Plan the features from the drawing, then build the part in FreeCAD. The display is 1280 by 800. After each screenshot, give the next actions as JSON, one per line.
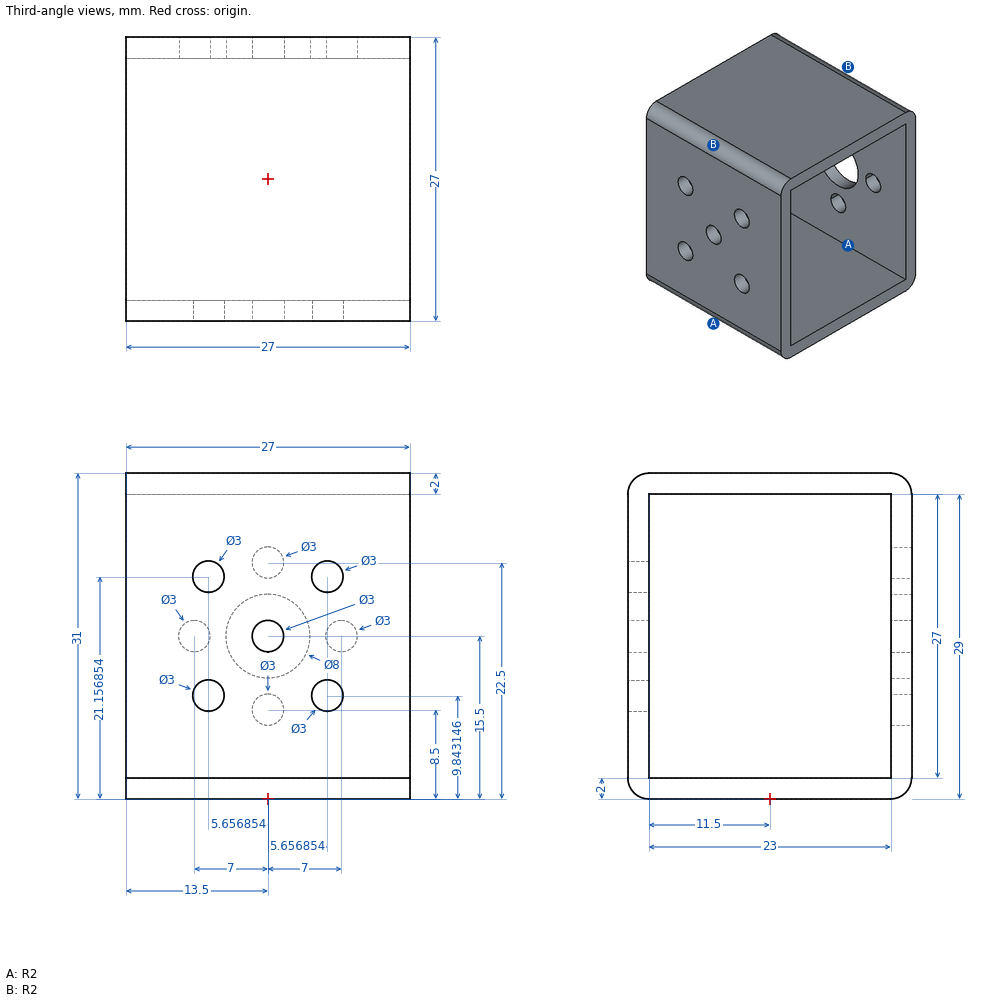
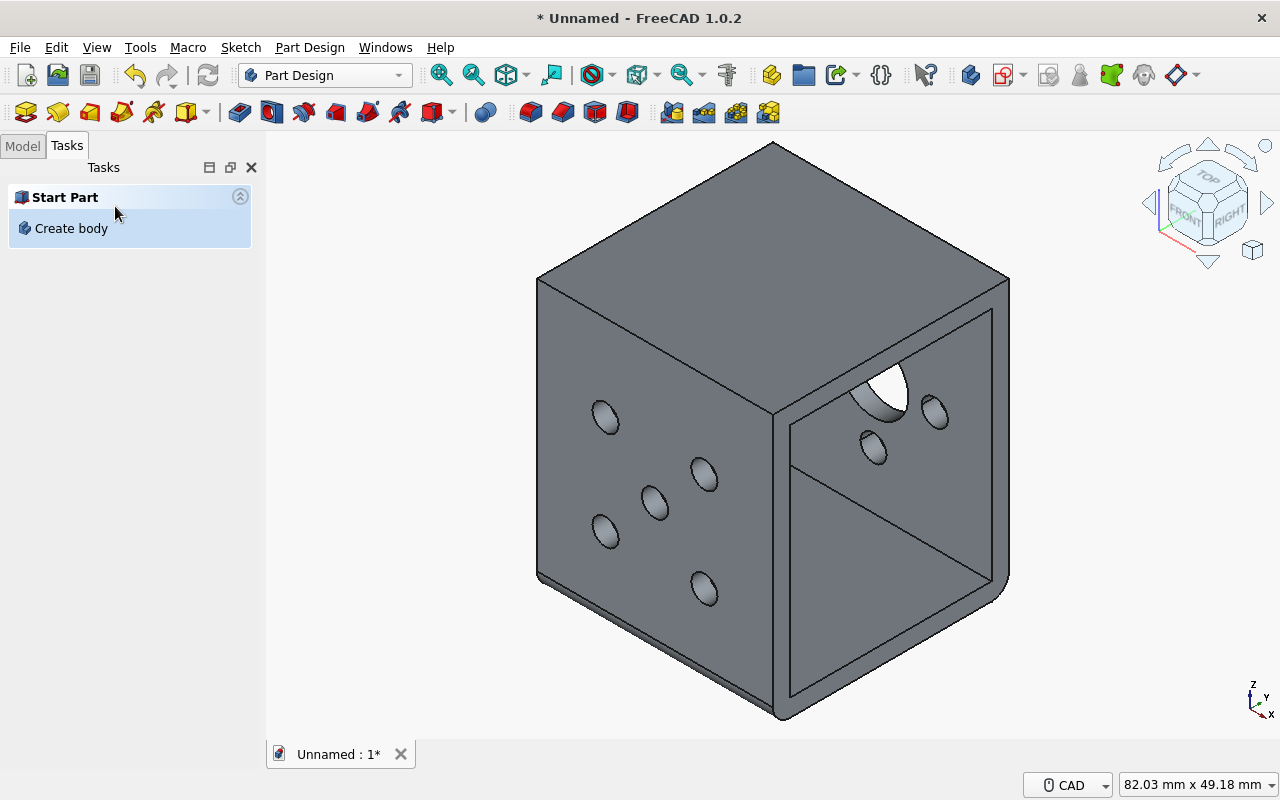
{"action": "left_click", "coordinate": [655, 346]}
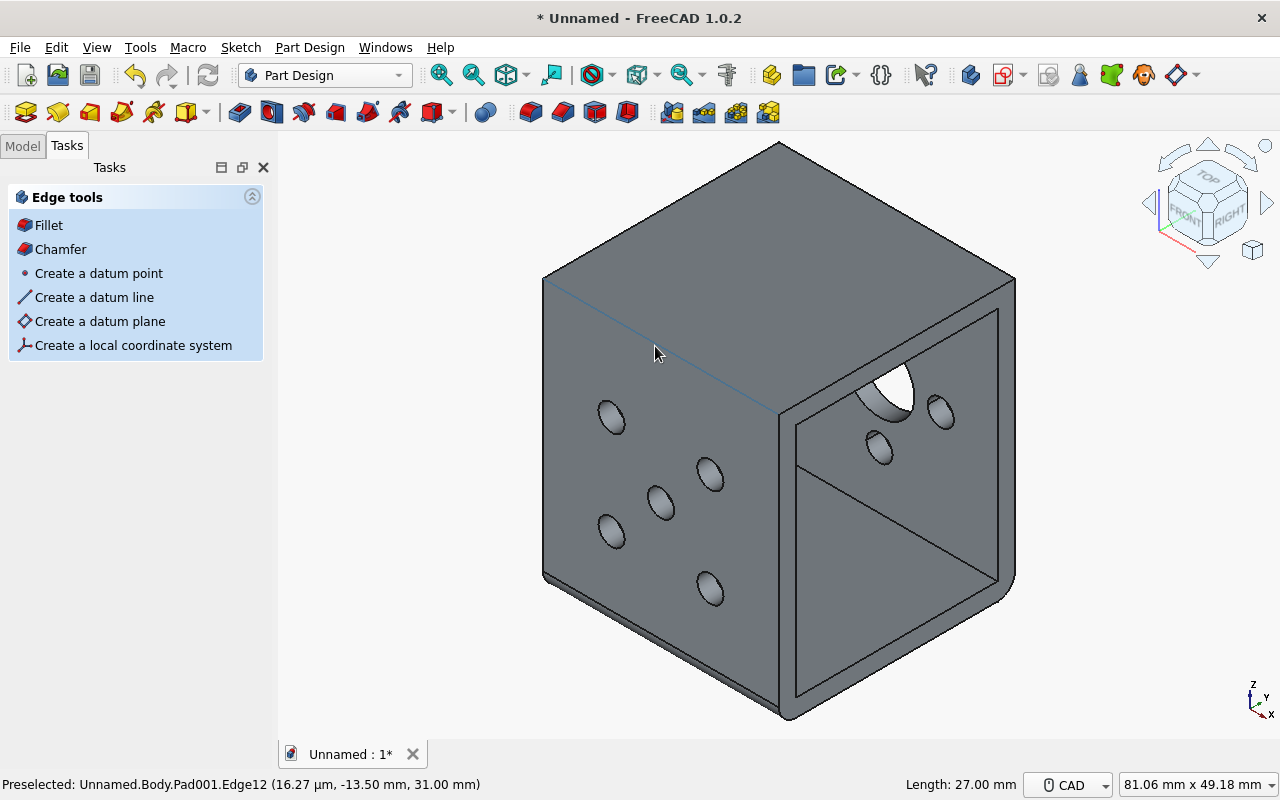
{"action": "key", "text": "2"}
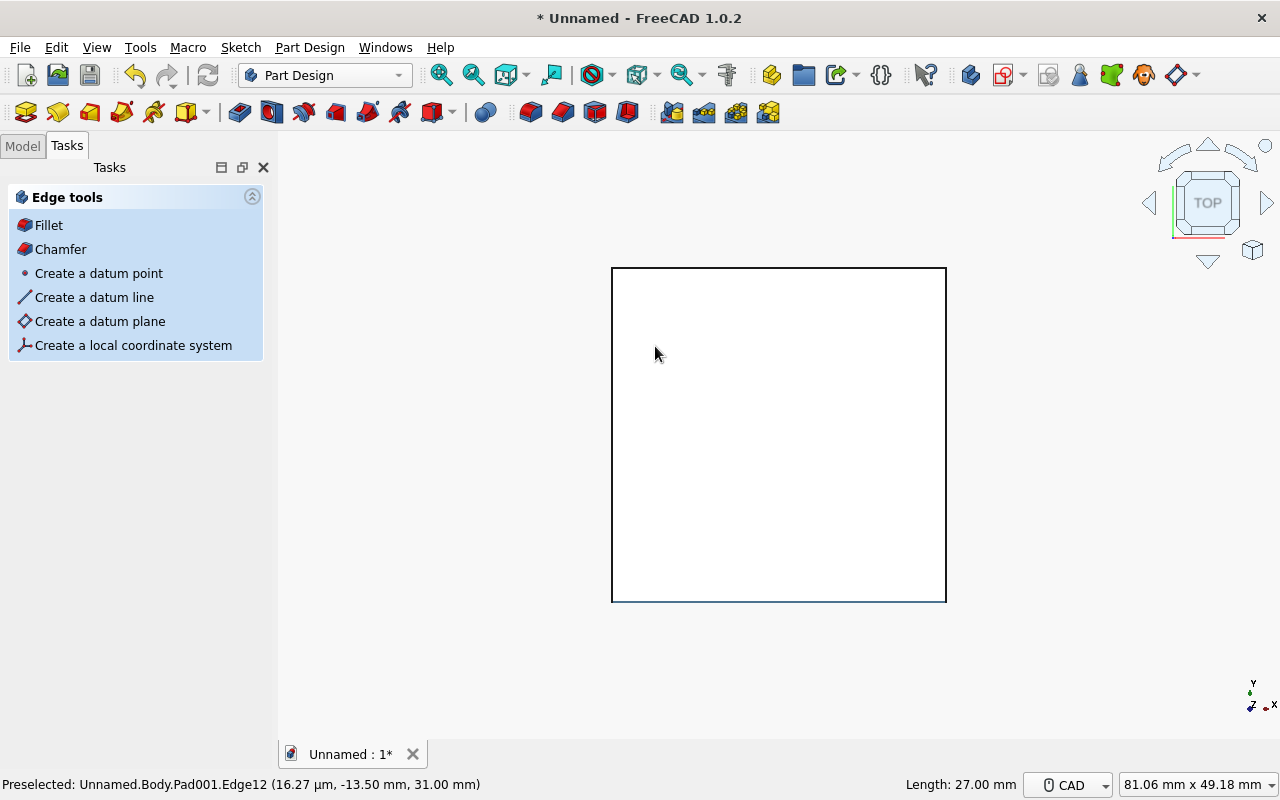
{"action": "left_click", "coordinate": [779, 267], "text": "ctrl"}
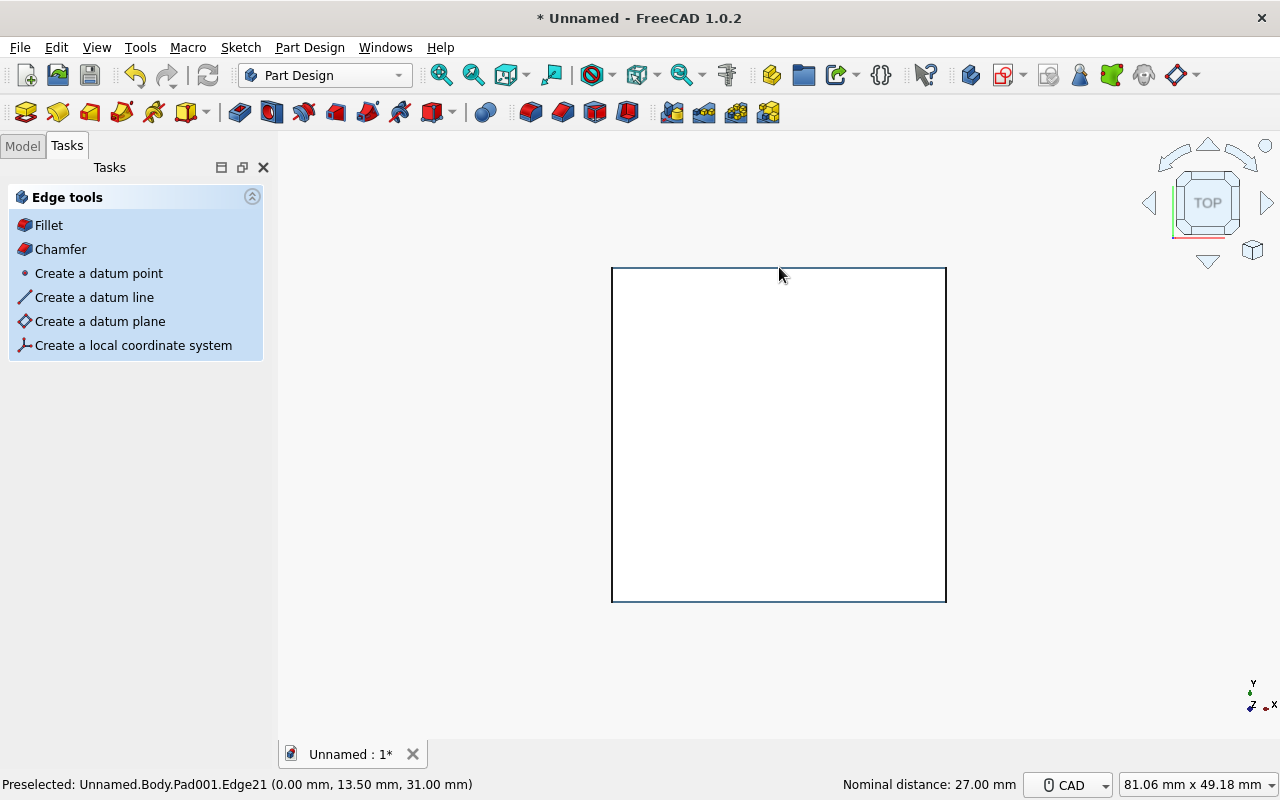
{"action": "left_click", "coordinate": [532, 112]}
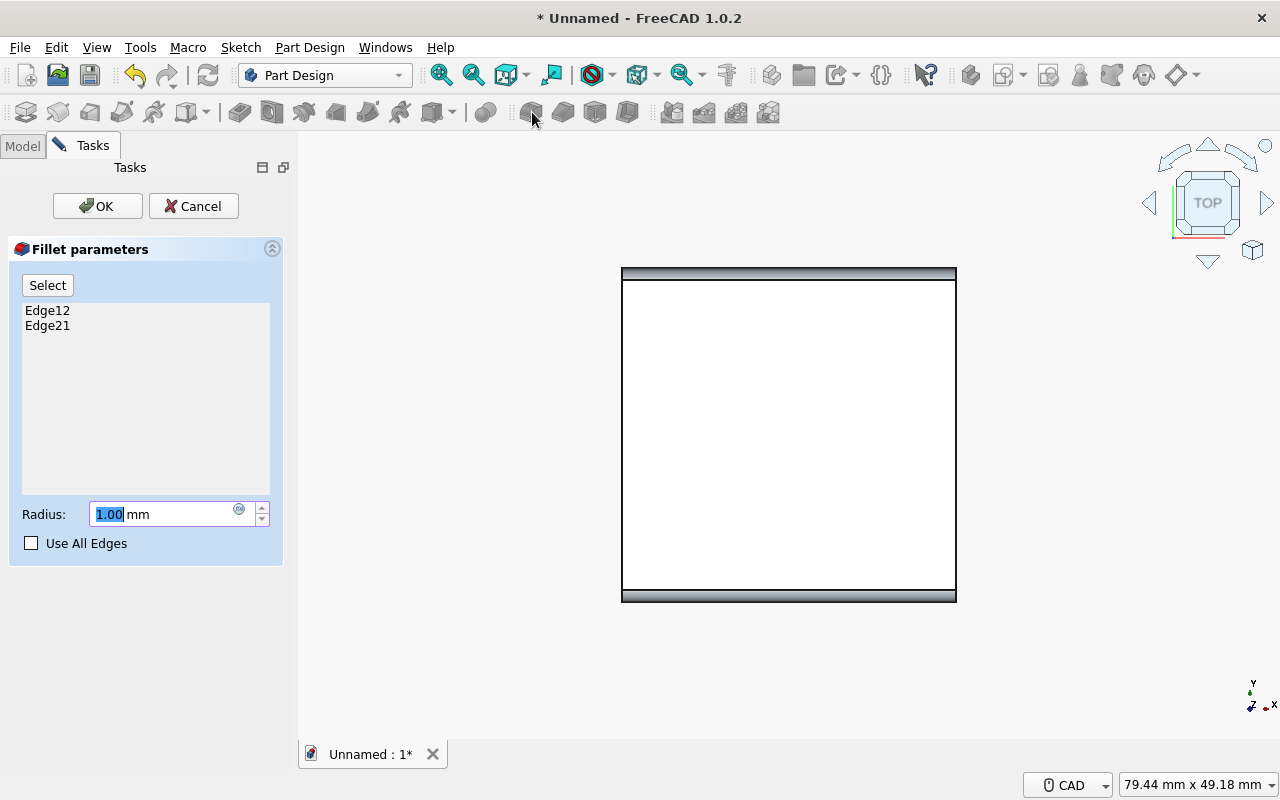
{"action": "type", "text": "2"}
{"action": "key", "text": "Tab"}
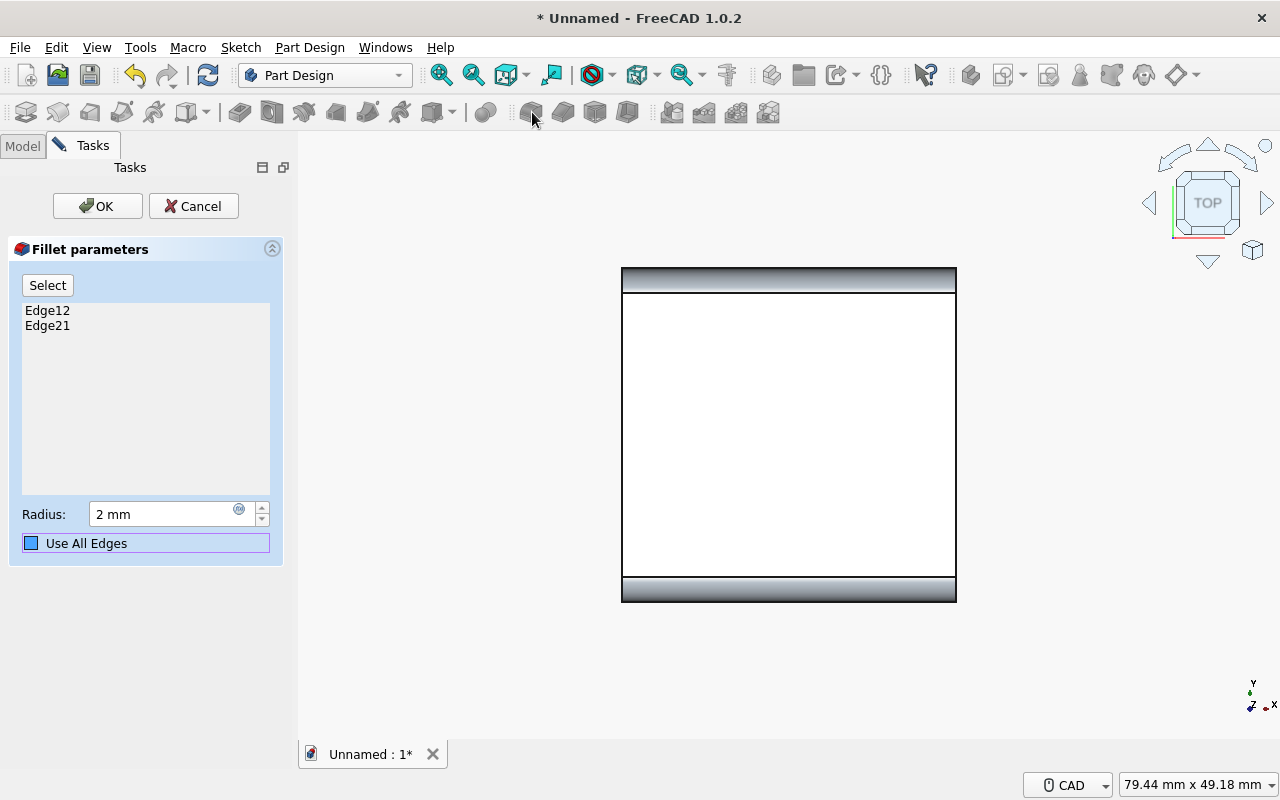
{"action": "left_click", "coordinate": [98, 206]}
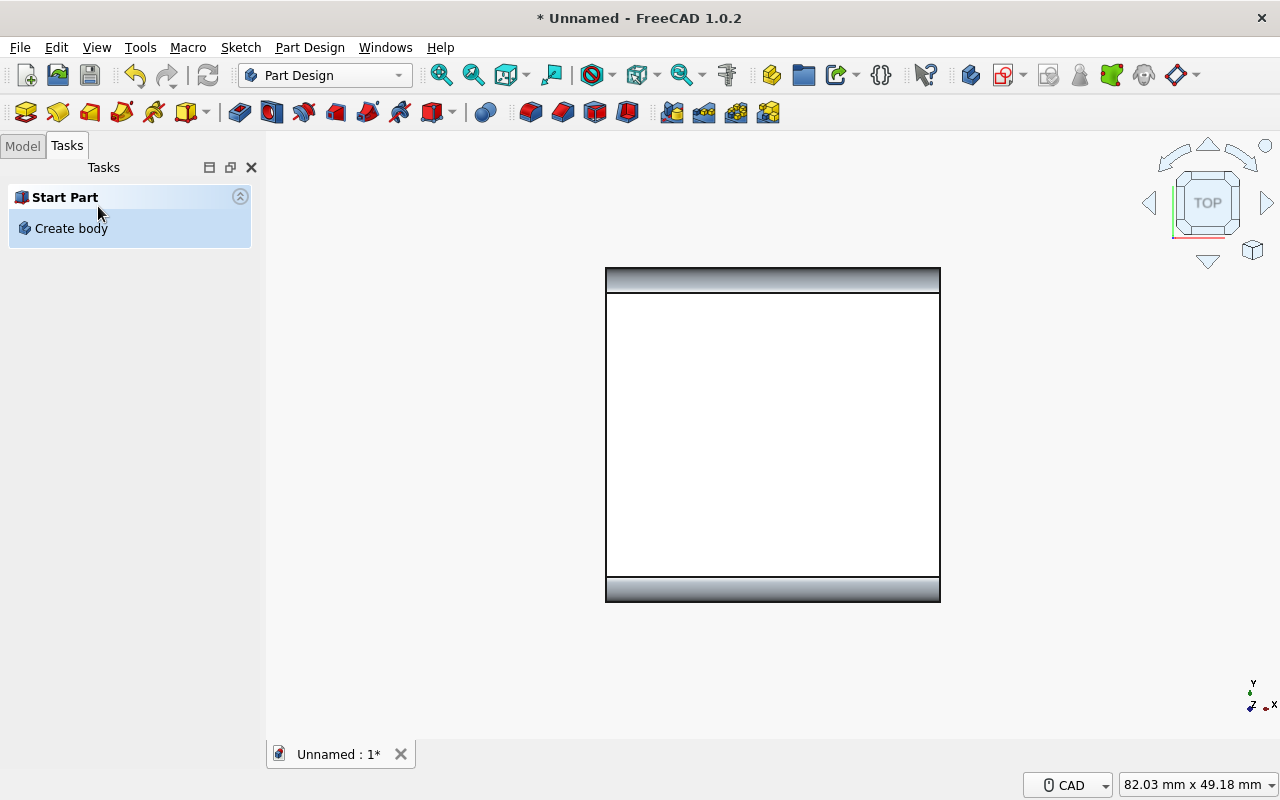
{"action": "key", "text": "0"}